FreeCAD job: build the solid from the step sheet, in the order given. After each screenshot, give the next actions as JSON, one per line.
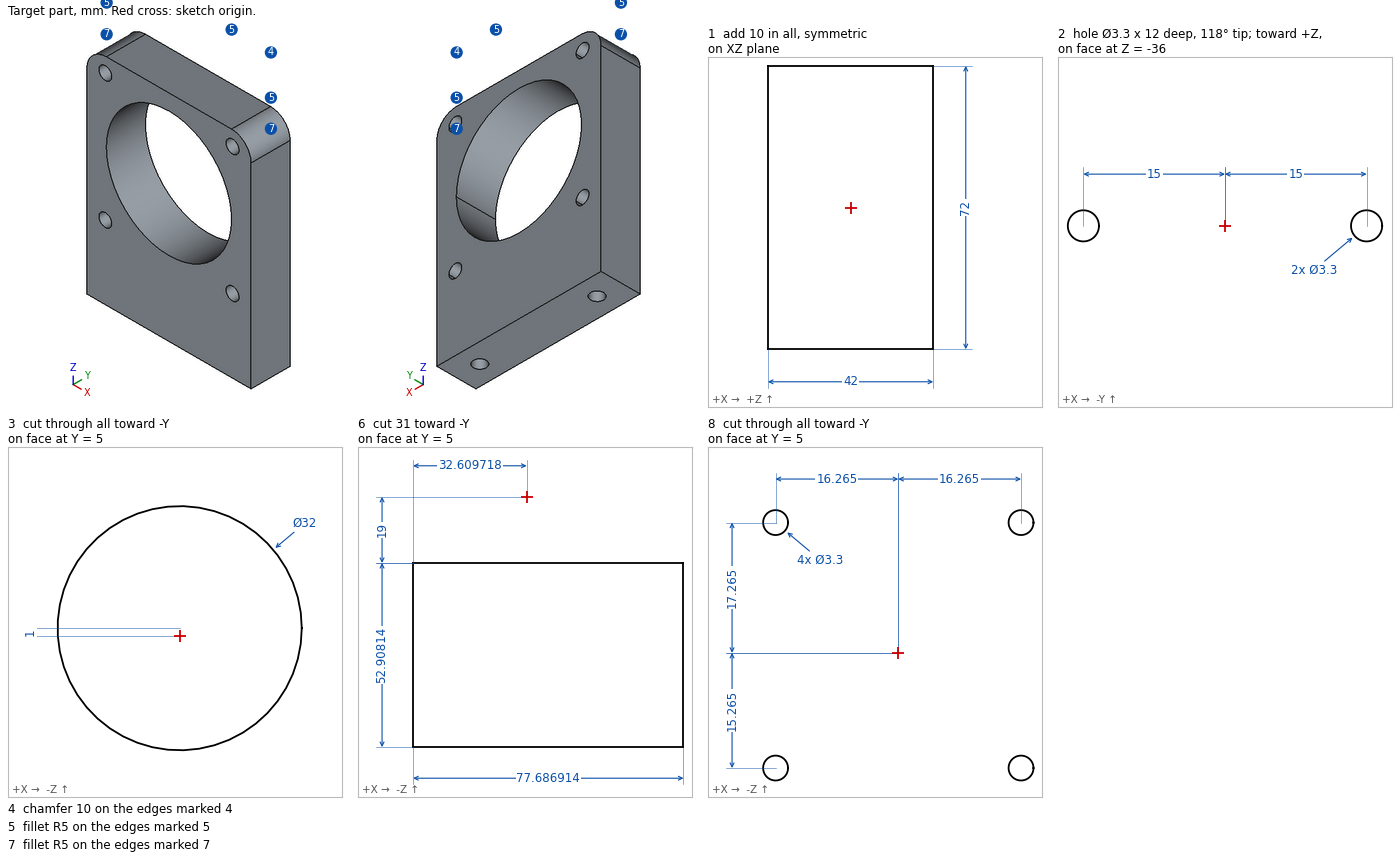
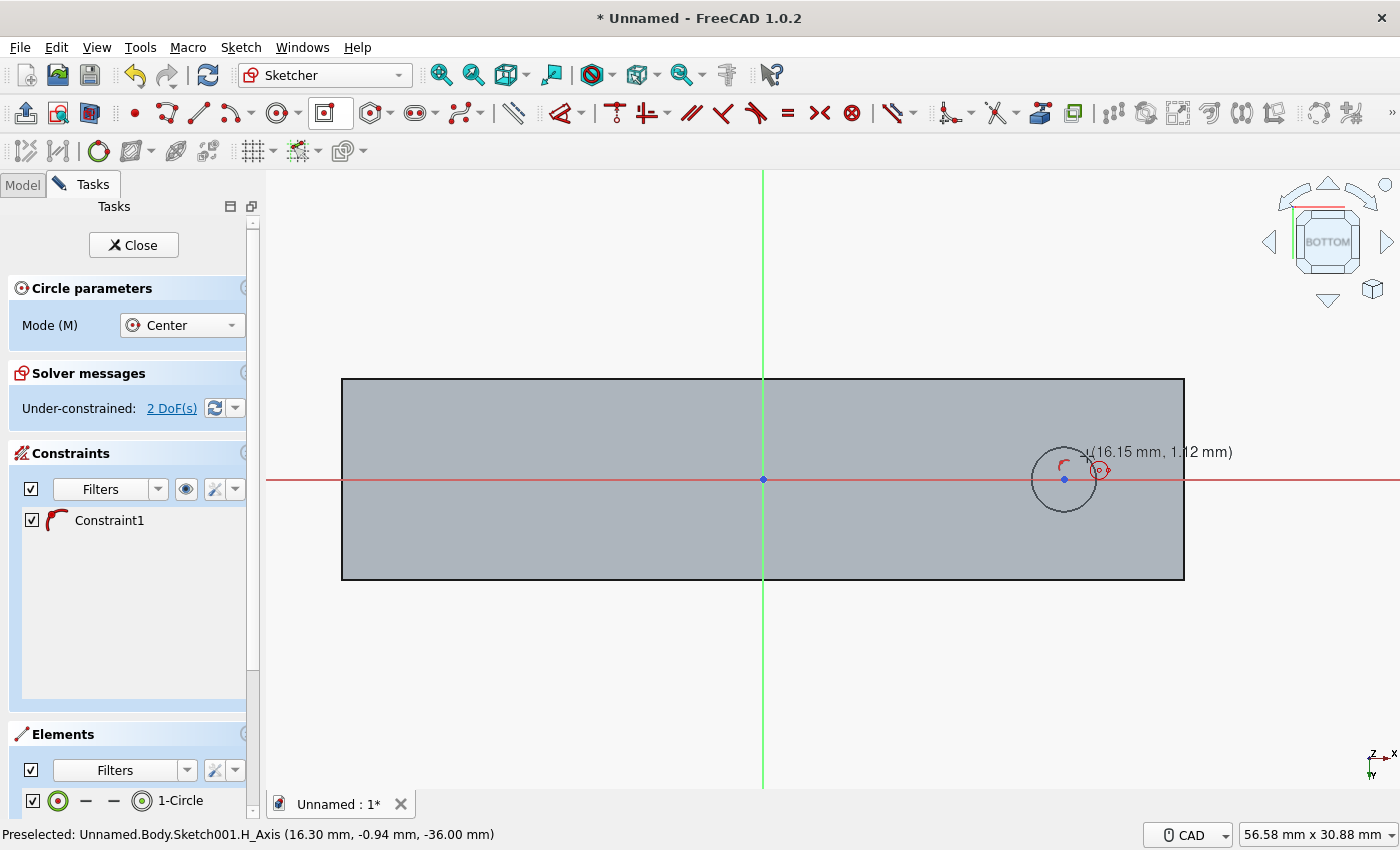
{"action": "left_click", "coordinate": [463, 479]}
{"action": "left_click", "coordinate": [486, 456]}
{"action": "key", "text": "Escape"}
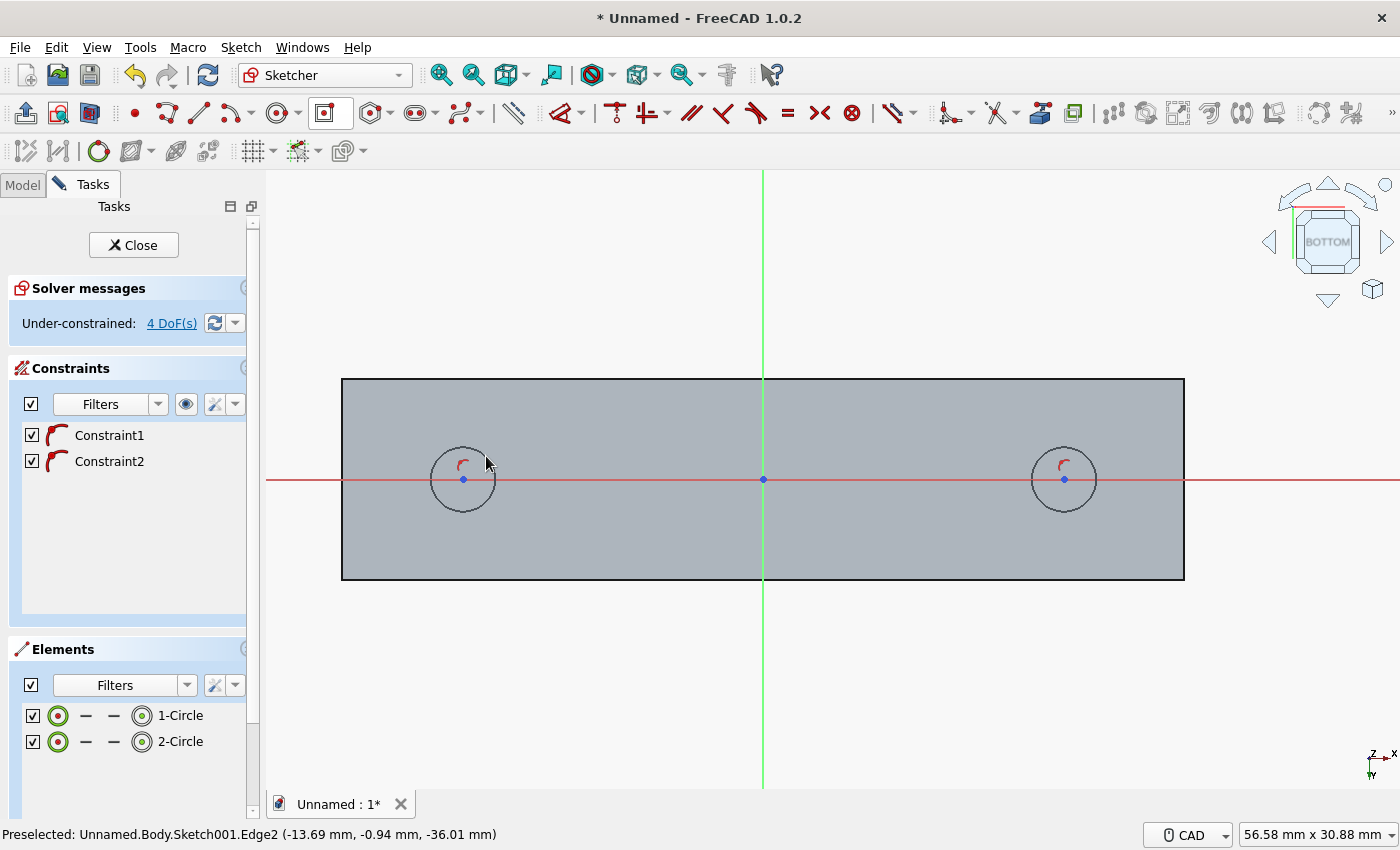
{"action": "left_click", "coordinate": [1087, 457]}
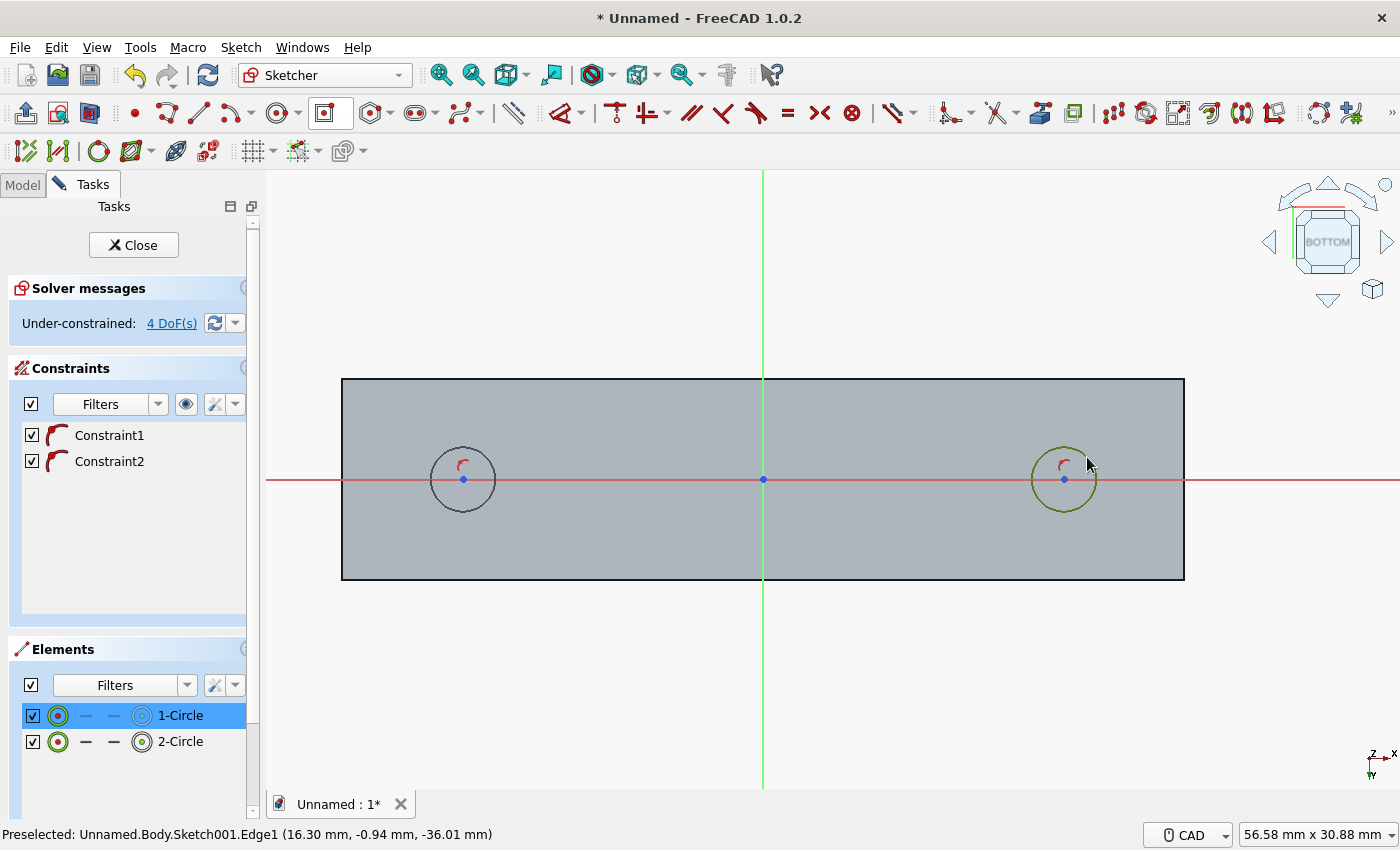
{"action": "left_click", "coordinate": [486, 457]}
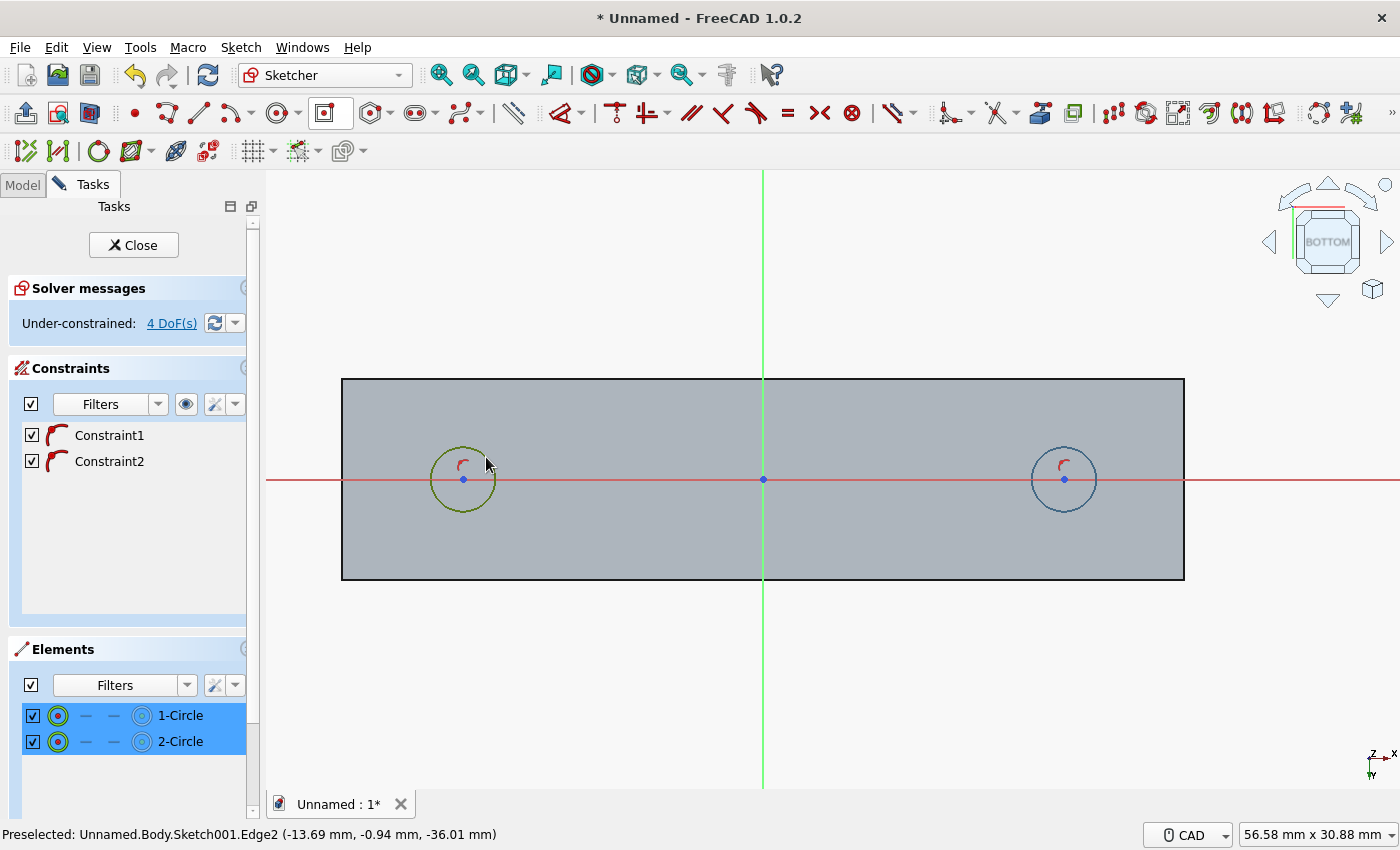
{"action": "key", "text": "e"}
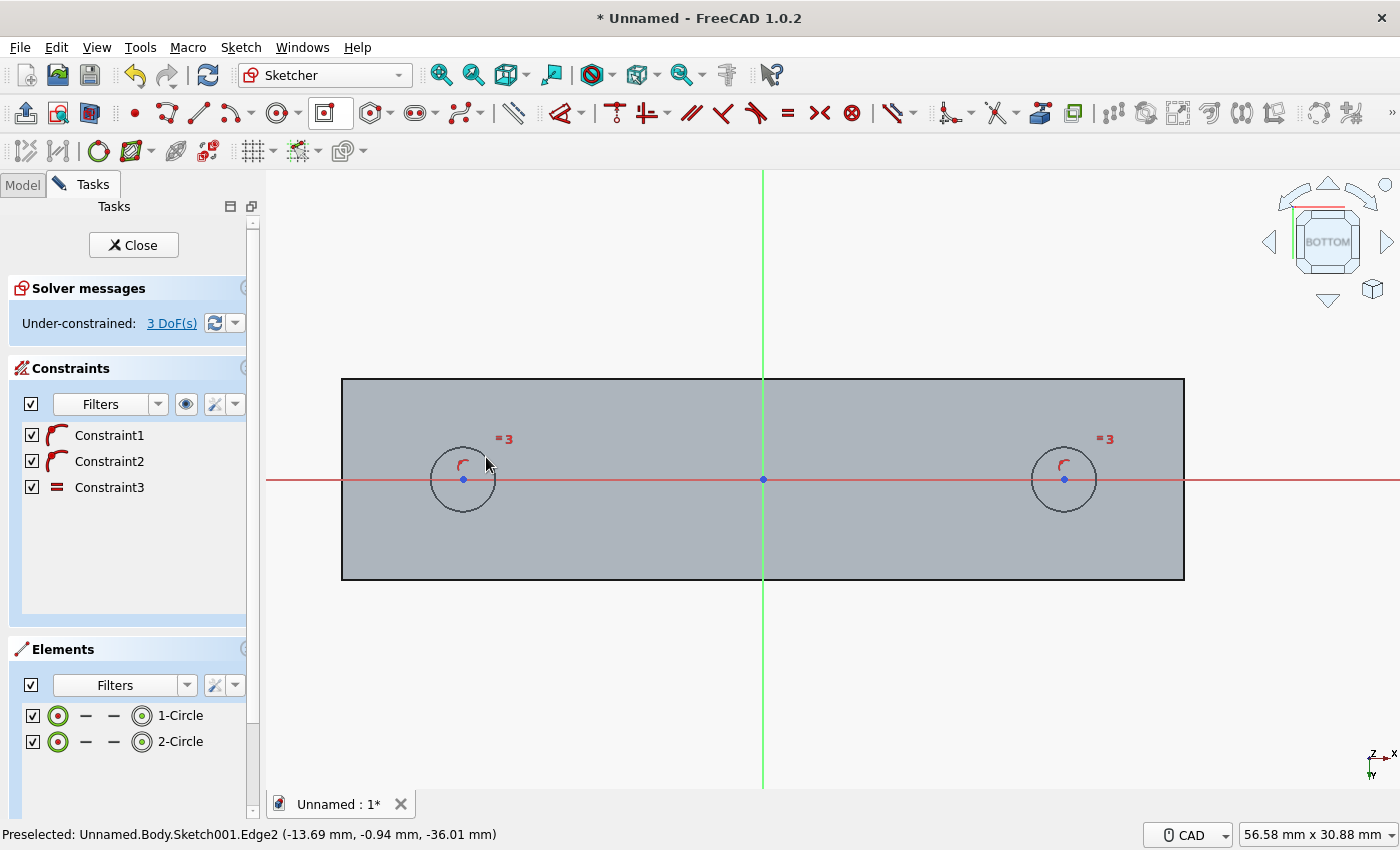
{"action": "left_click", "coordinate": [560, 114]}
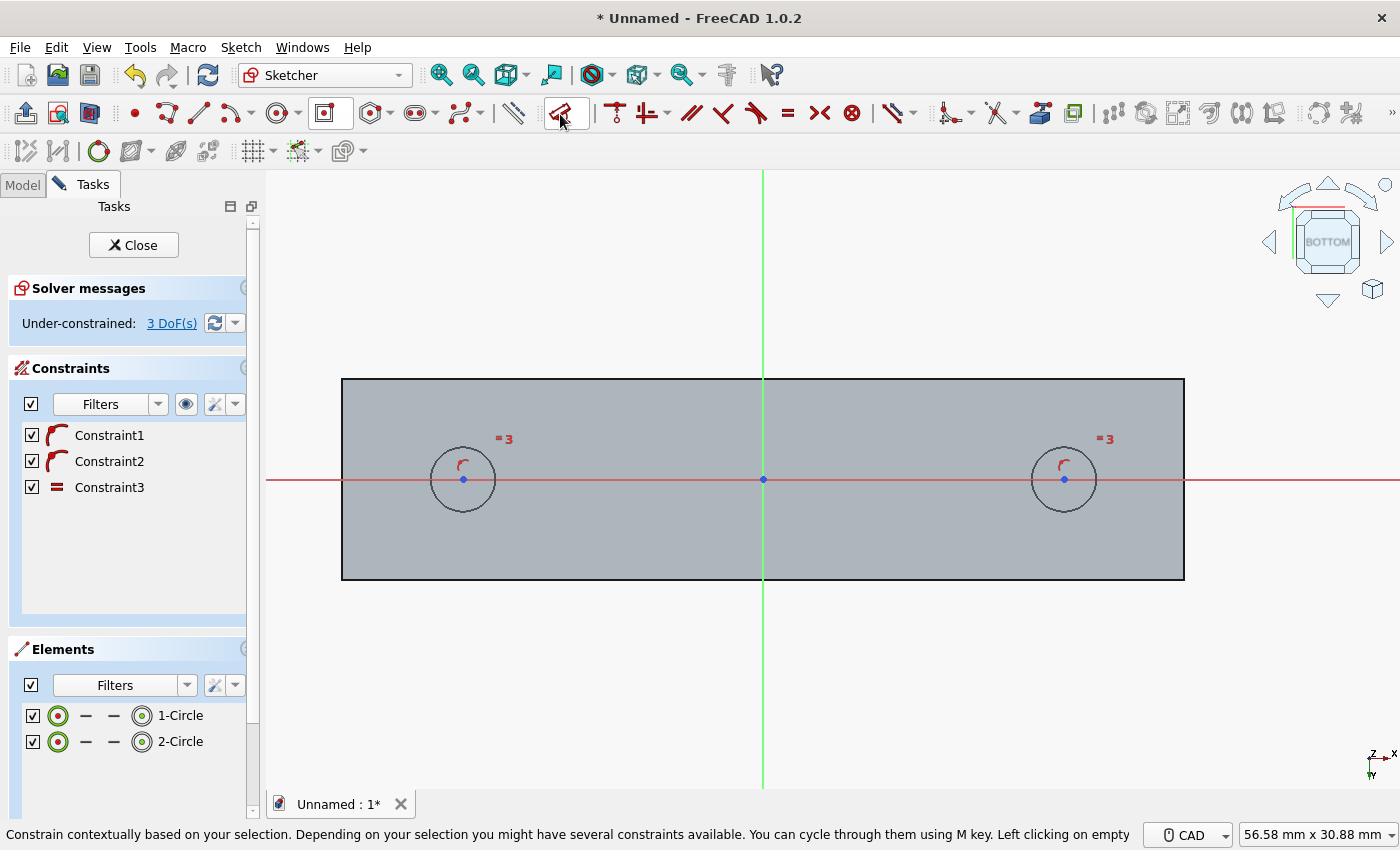
{"action": "left_click", "coordinate": [1087, 457]}
{"action": "left_click", "coordinate": [1110, 435]}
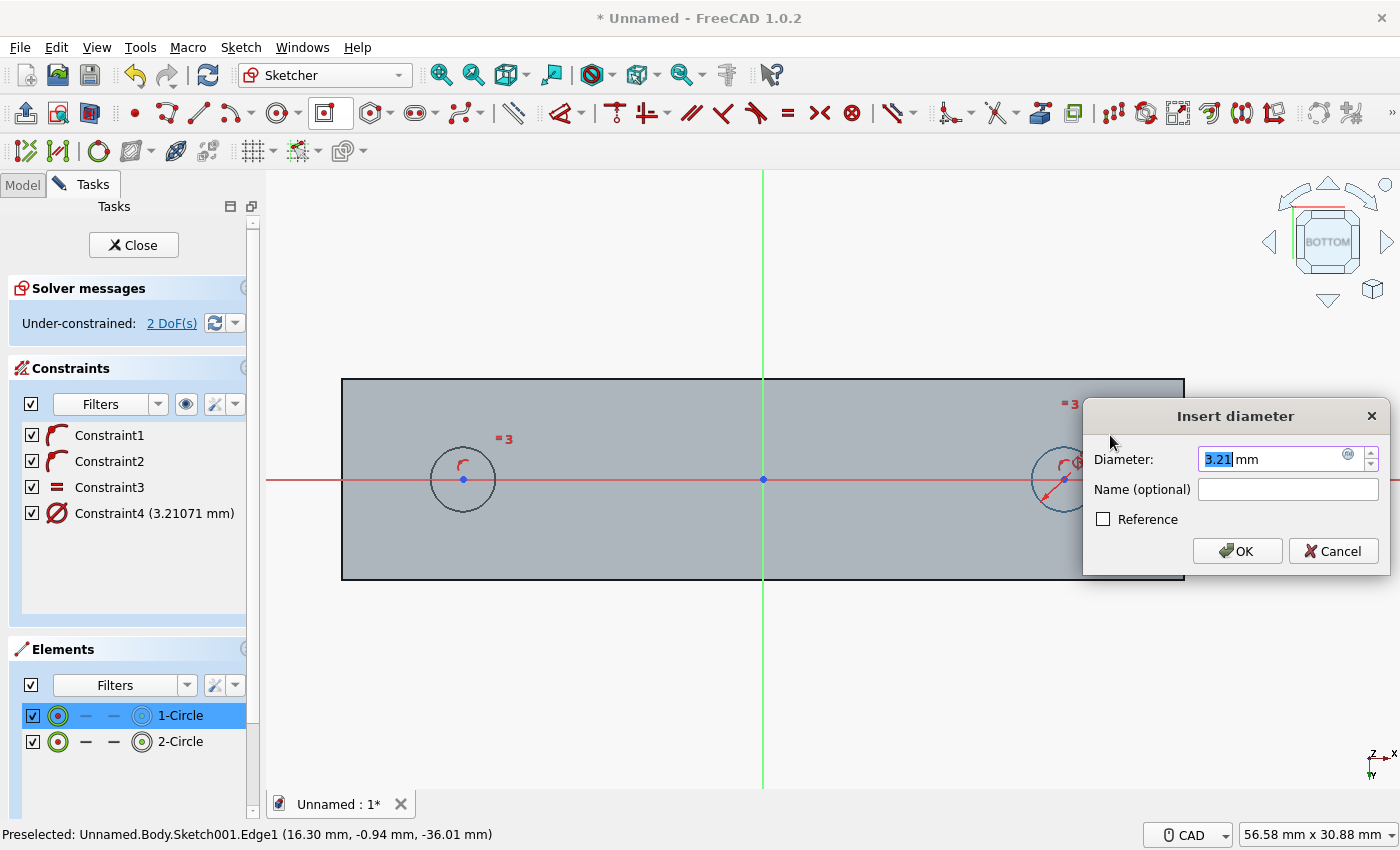
{"action": "type", "text": "3.3"}
{"action": "key", "text": "Return"}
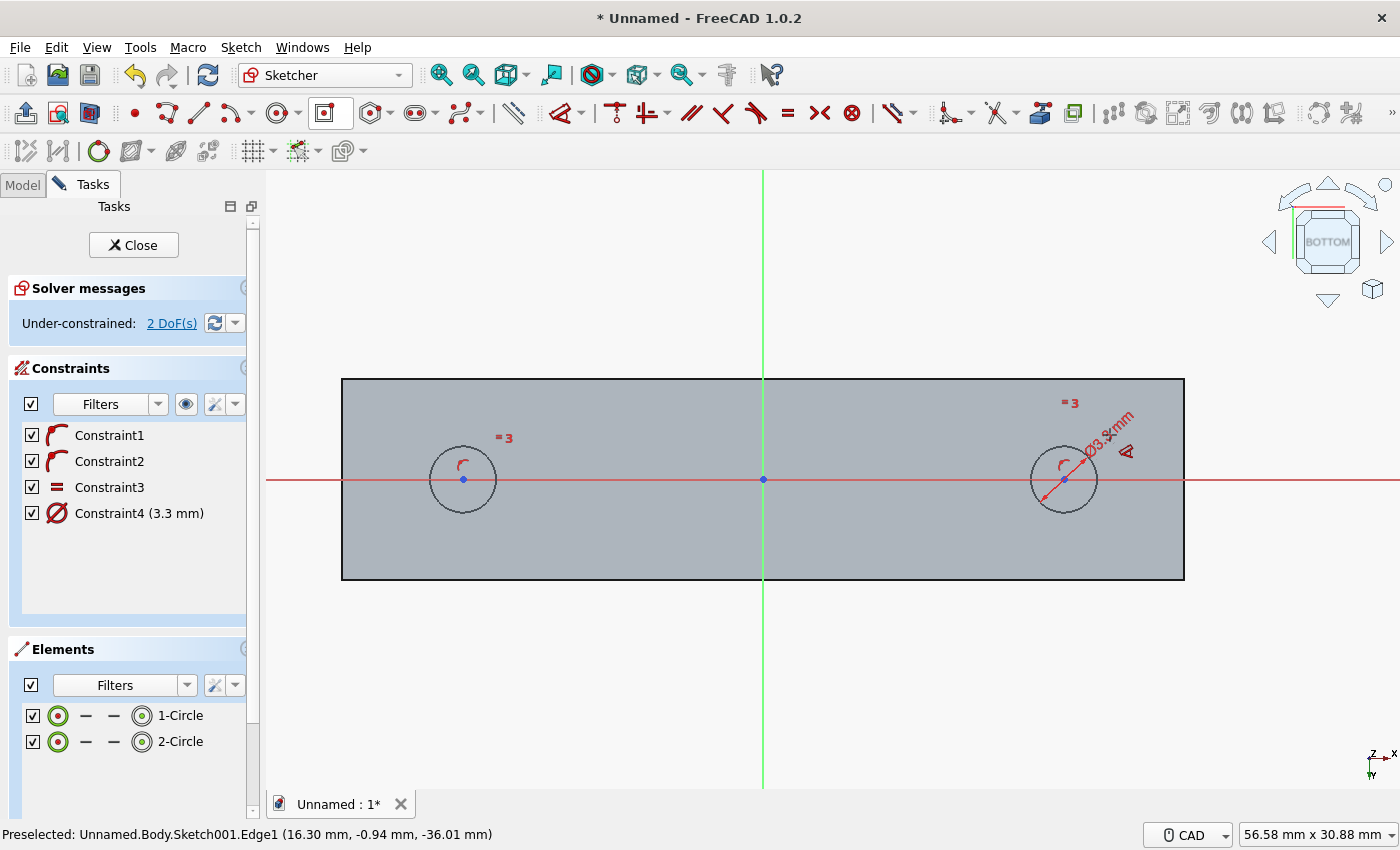
{"action": "left_click", "coordinate": [1064, 479]}
{"action": "left_click", "coordinate": [914, 513]}